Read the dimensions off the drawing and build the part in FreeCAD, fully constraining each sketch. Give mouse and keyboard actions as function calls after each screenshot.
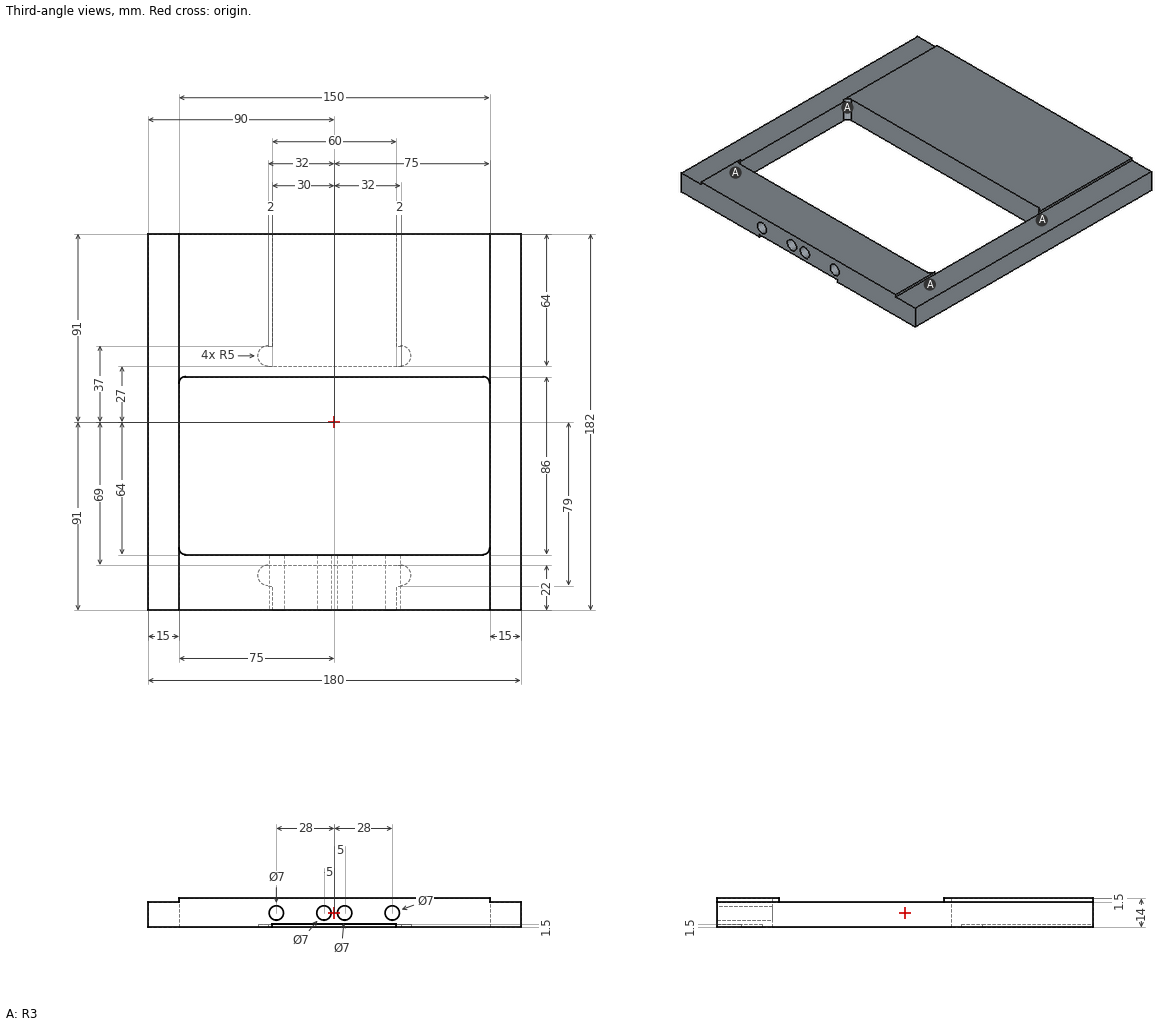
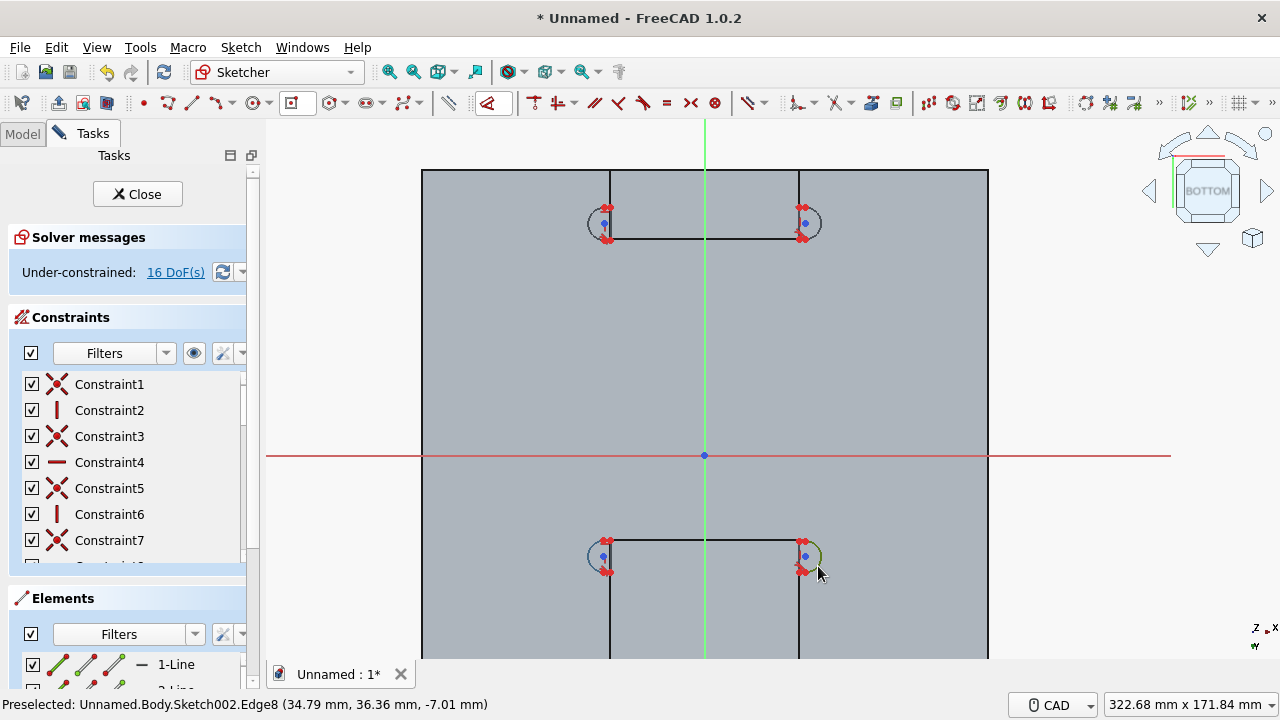
click(591, 214)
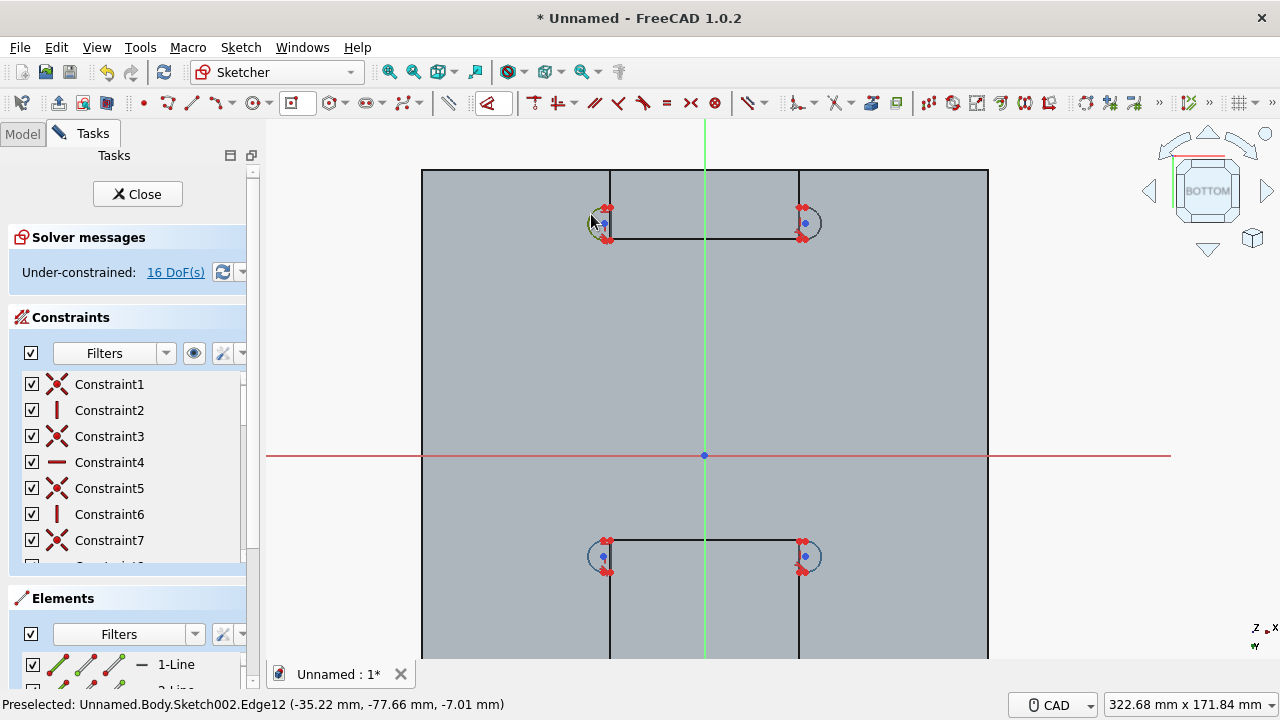
click(818, 233)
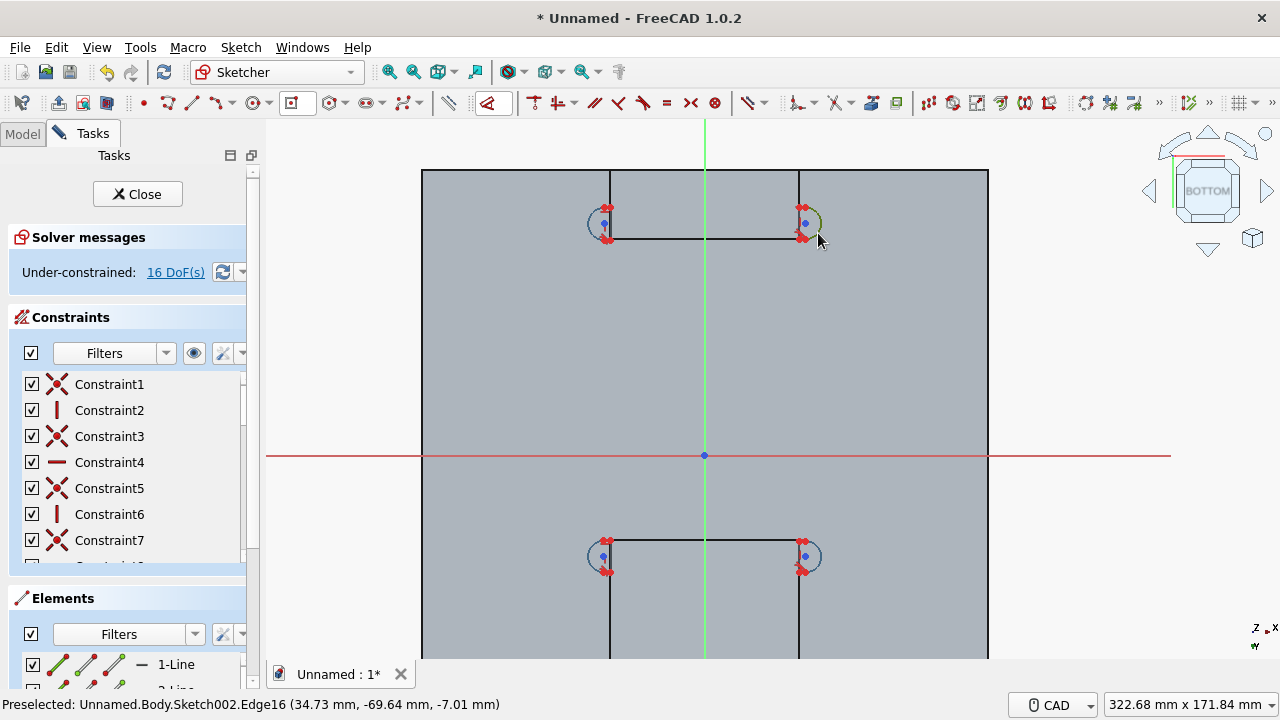
key(e)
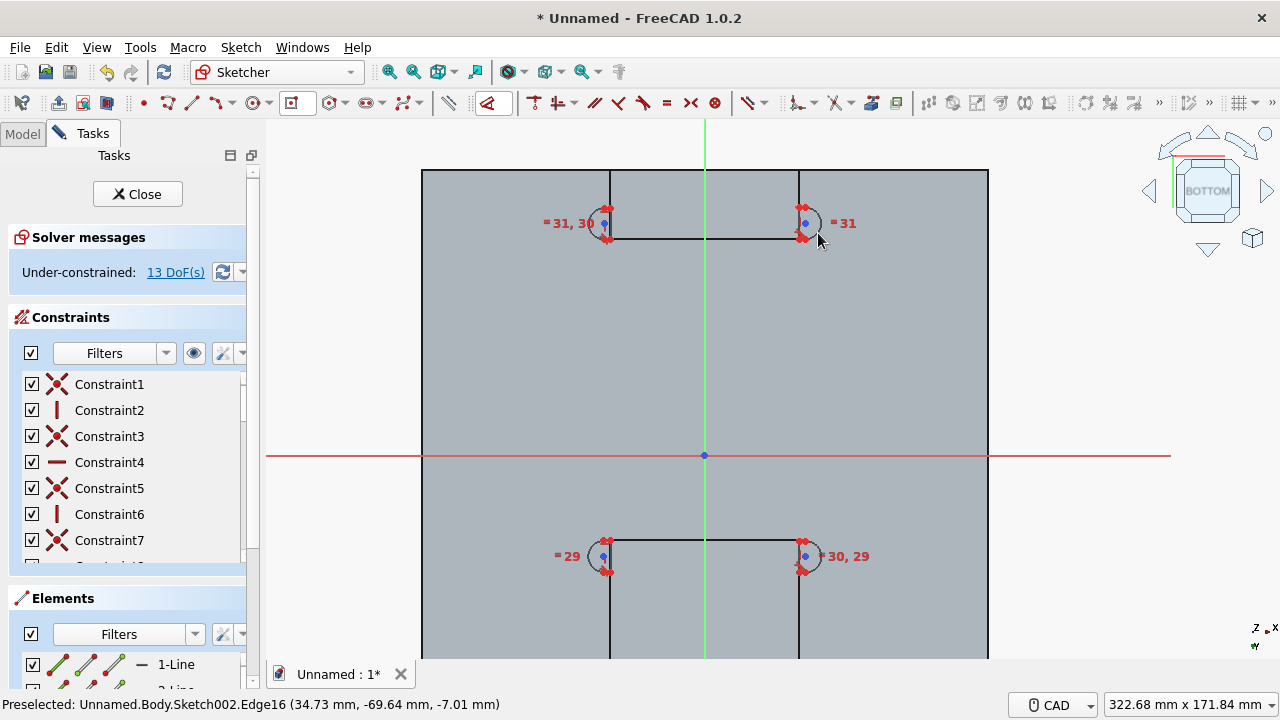
scroll(591, 547, up, 5)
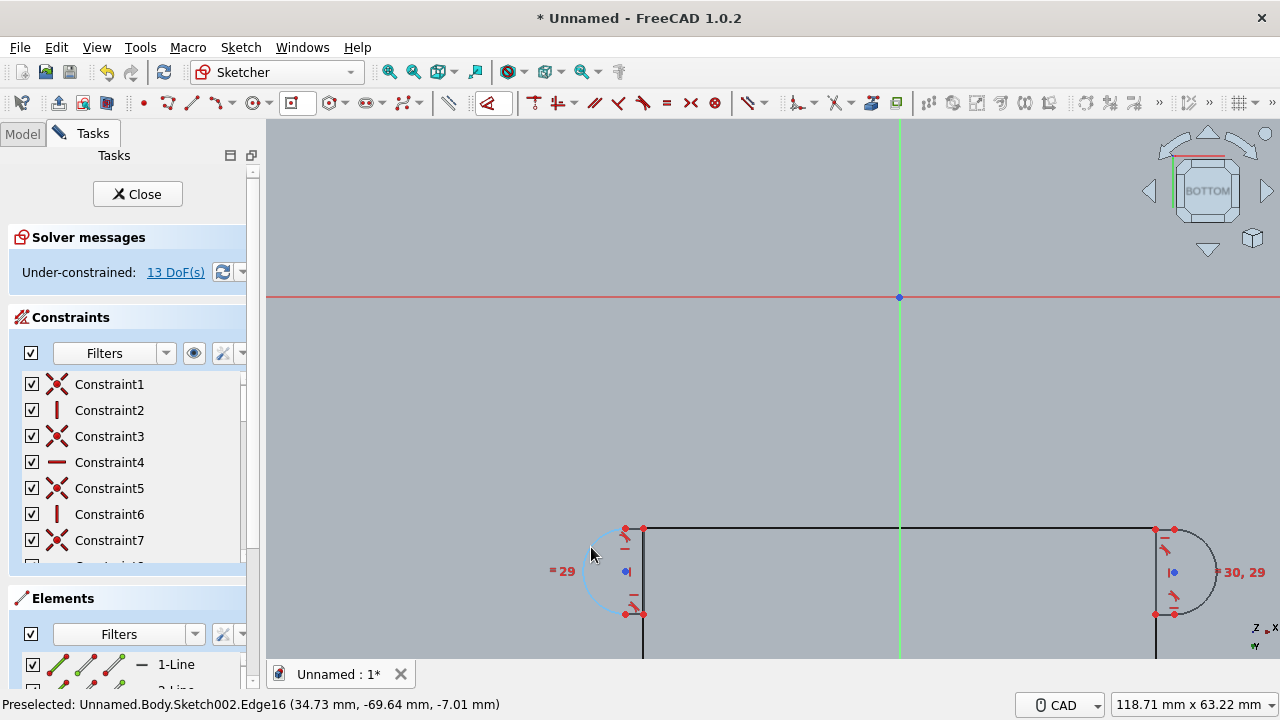
click(591, 546)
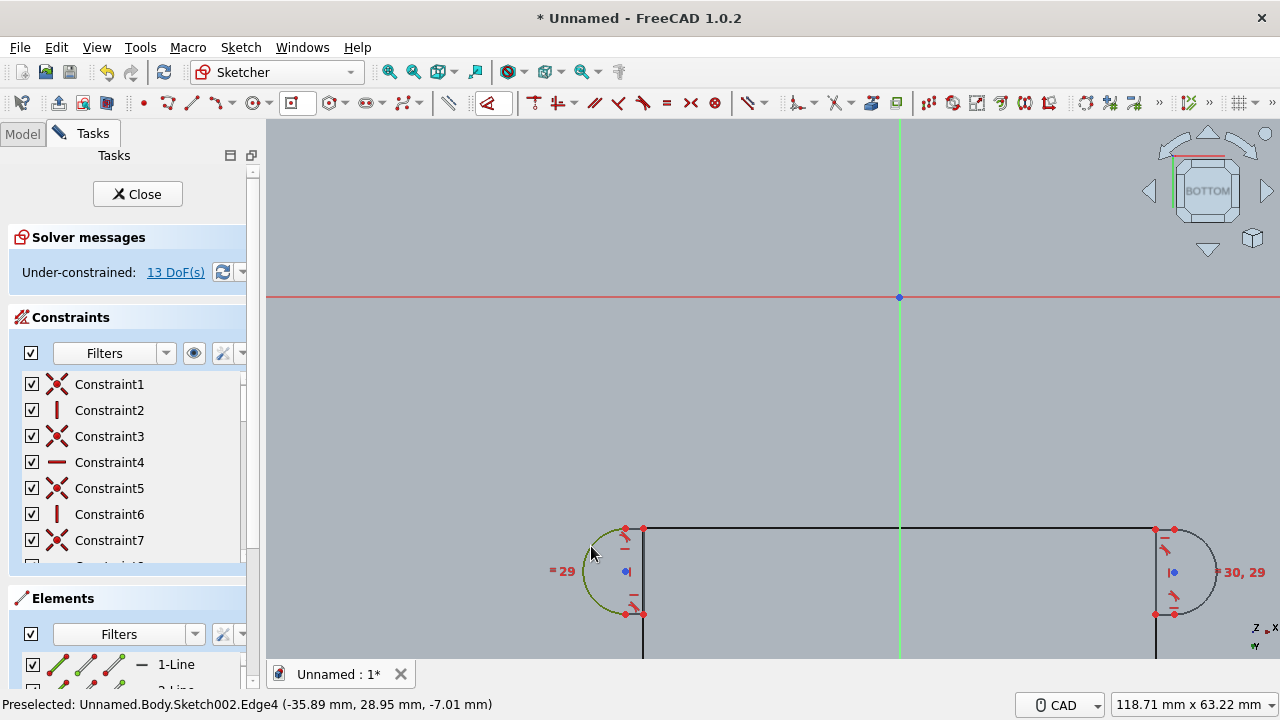
click(506, 104)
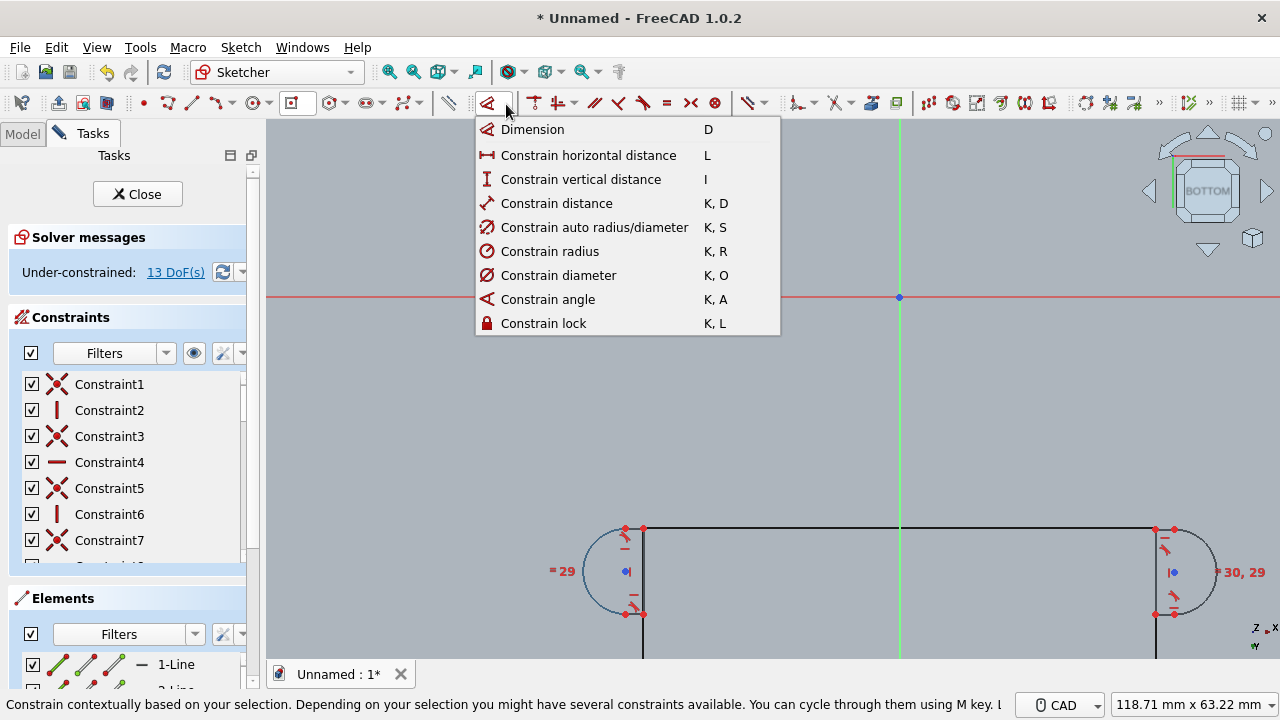
click(628, 251)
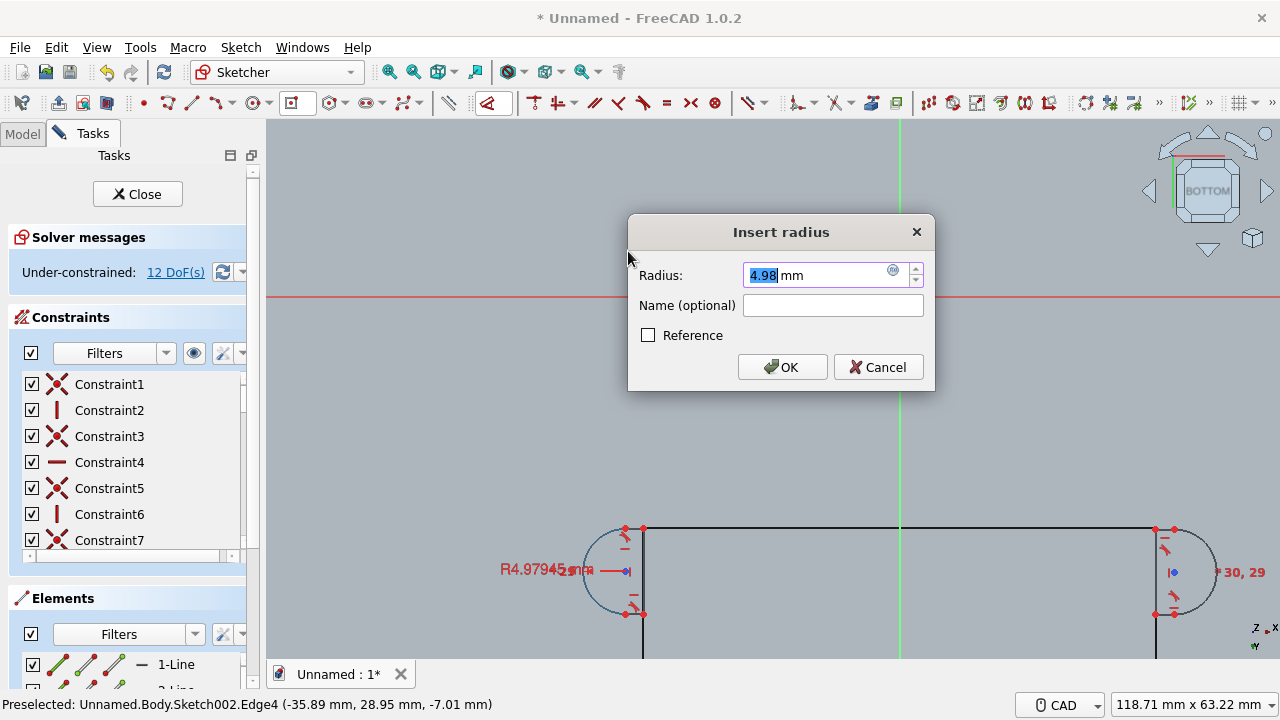
text(5)
key(Return)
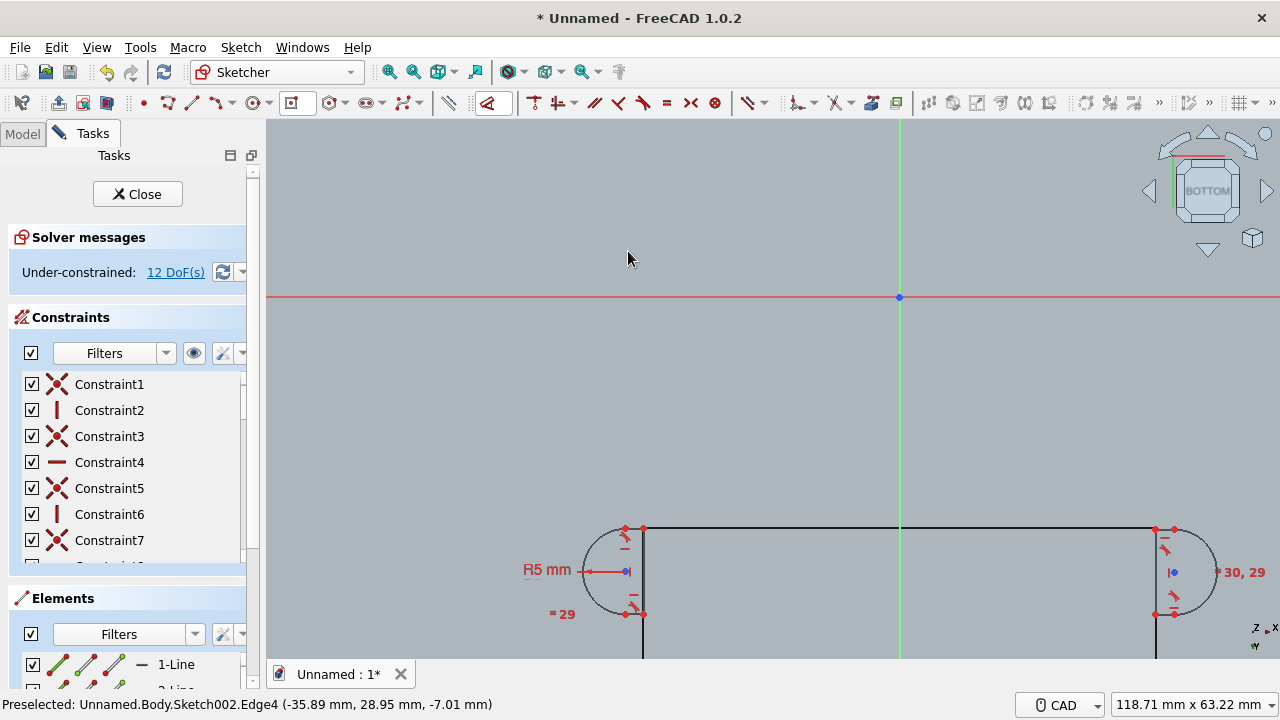
scroll(635, 614, up, 5)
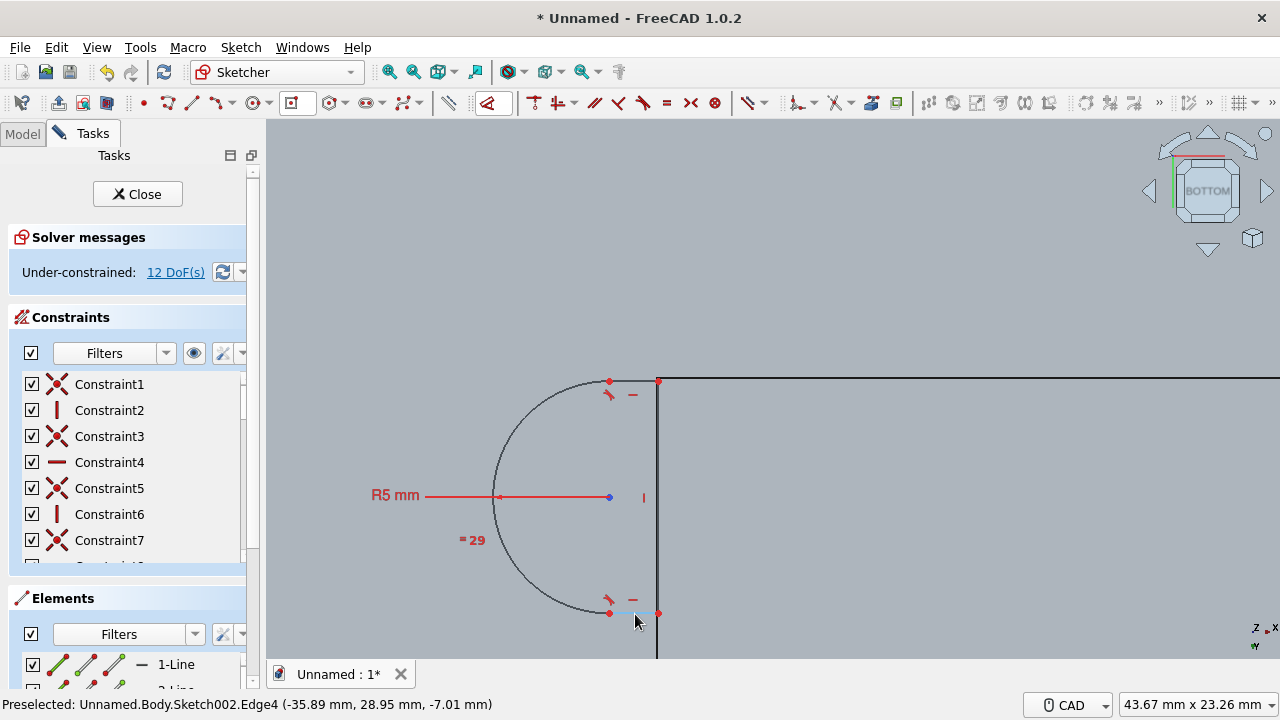
click(634, 613)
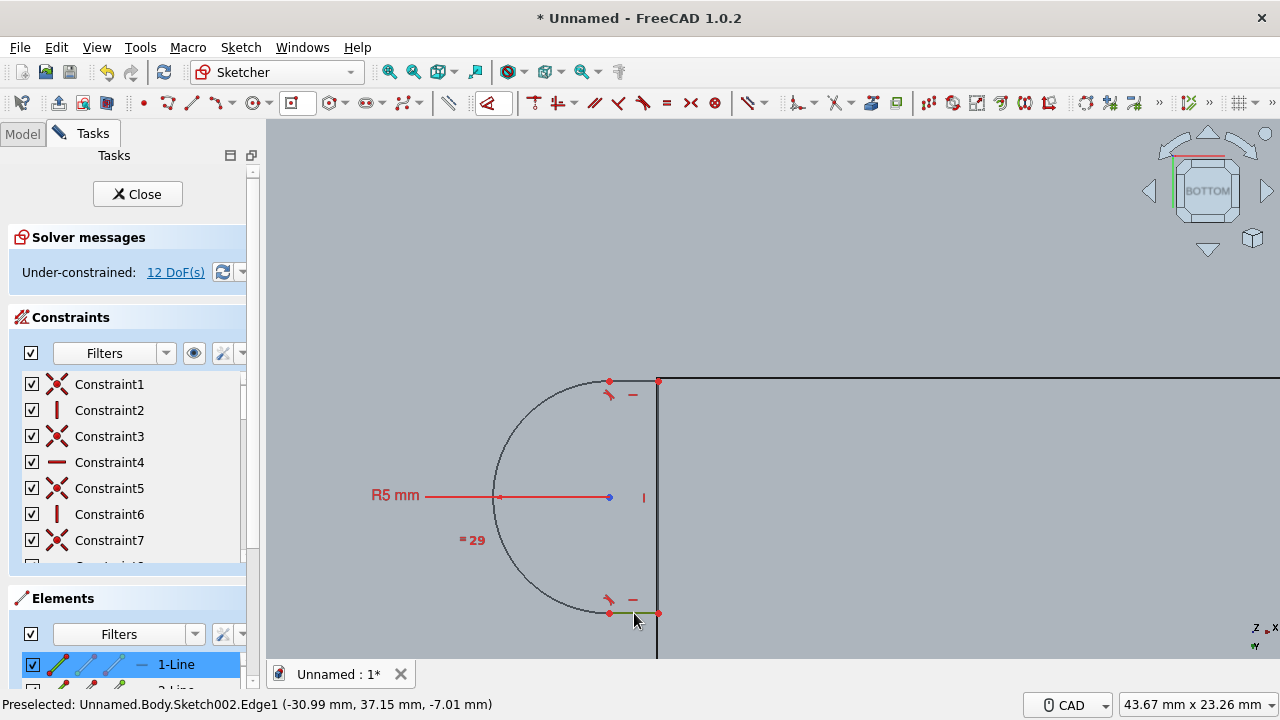
key(l)